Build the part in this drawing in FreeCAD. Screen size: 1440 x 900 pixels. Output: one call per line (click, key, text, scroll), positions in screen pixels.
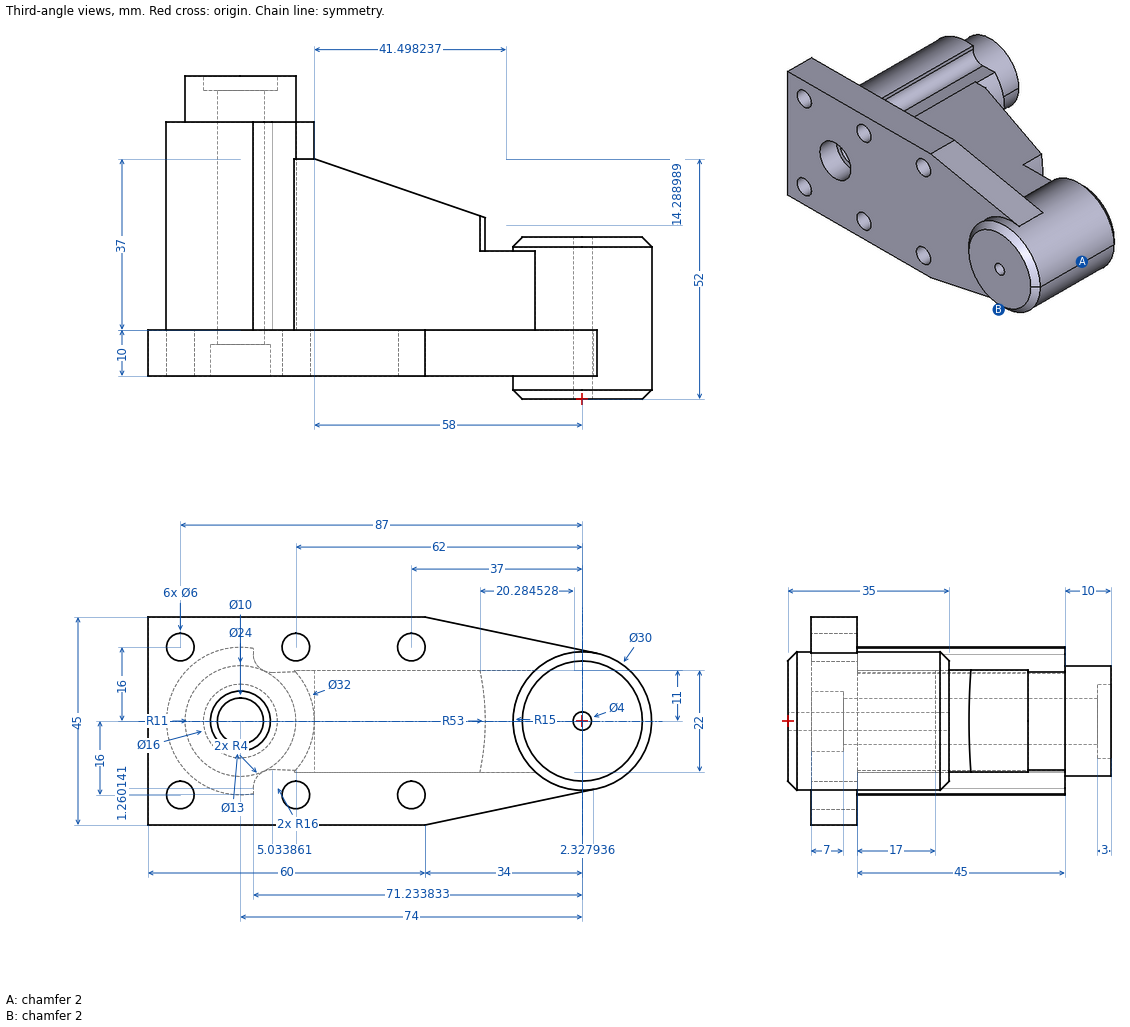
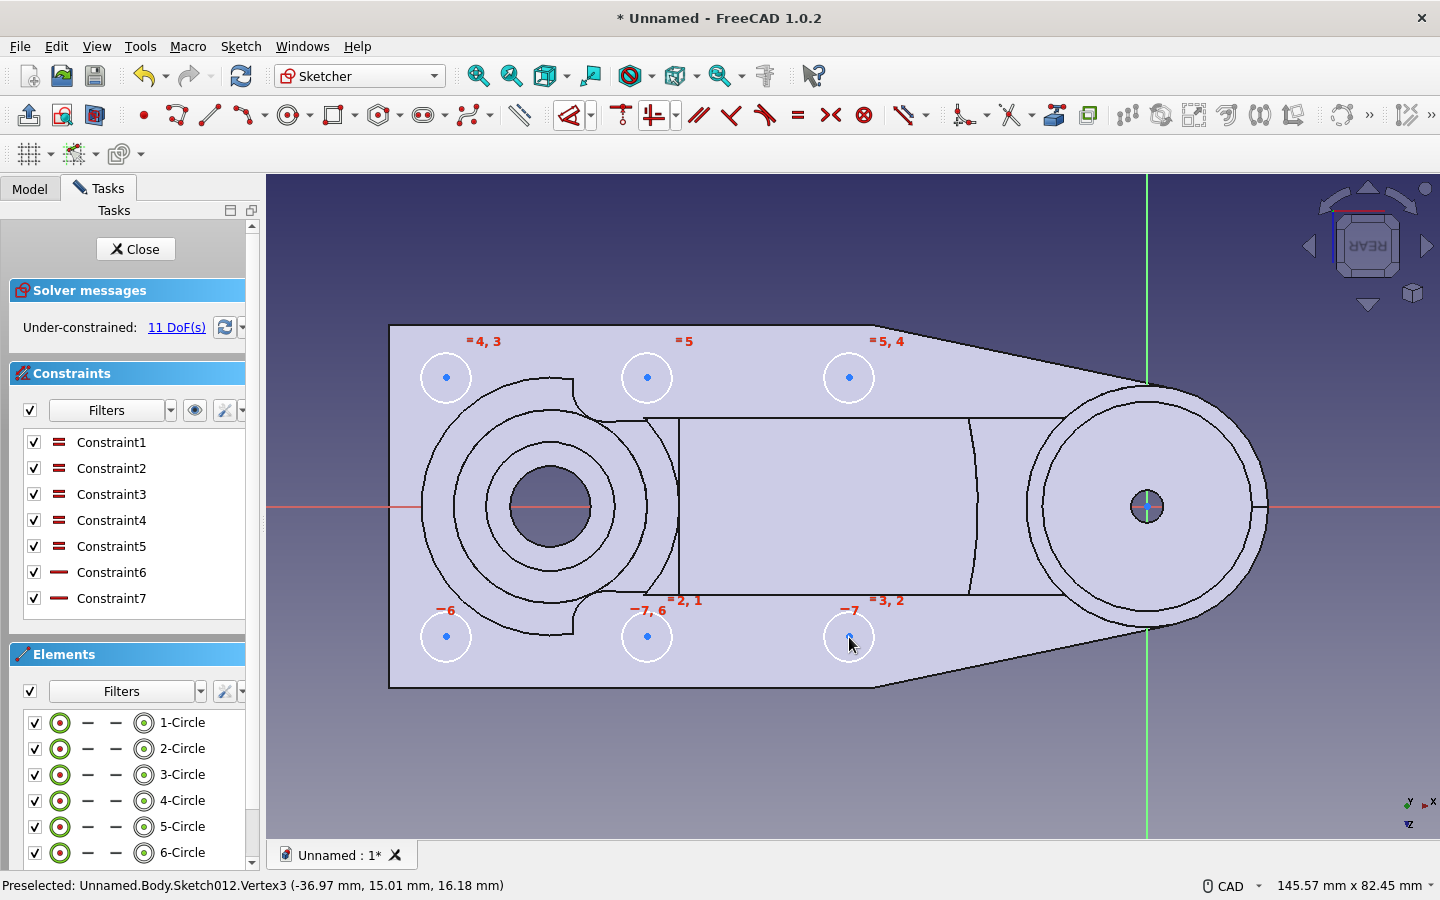
click(446, 637)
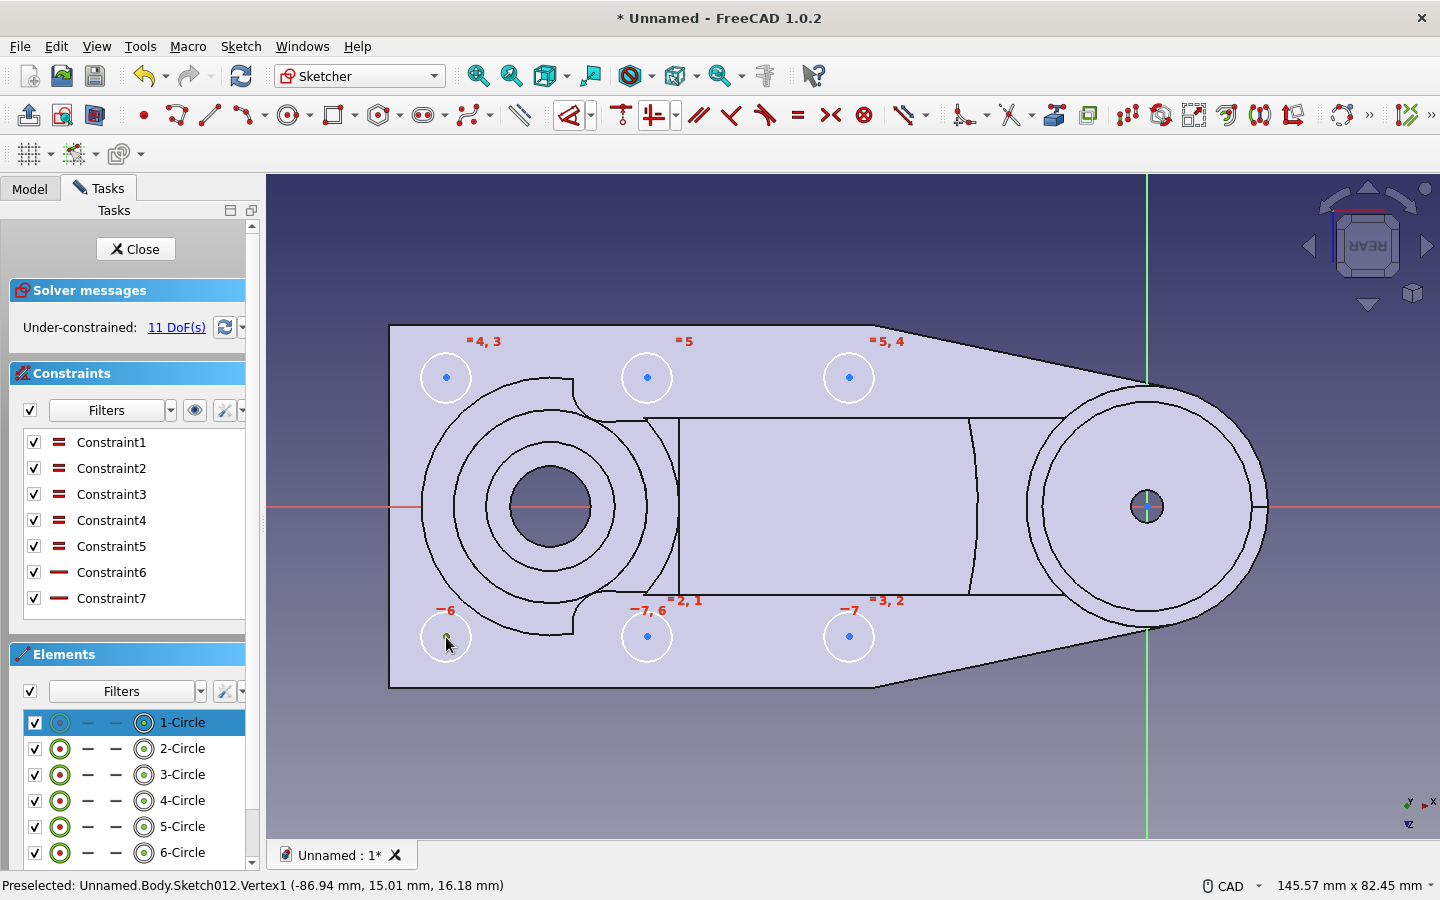
click(446, 378)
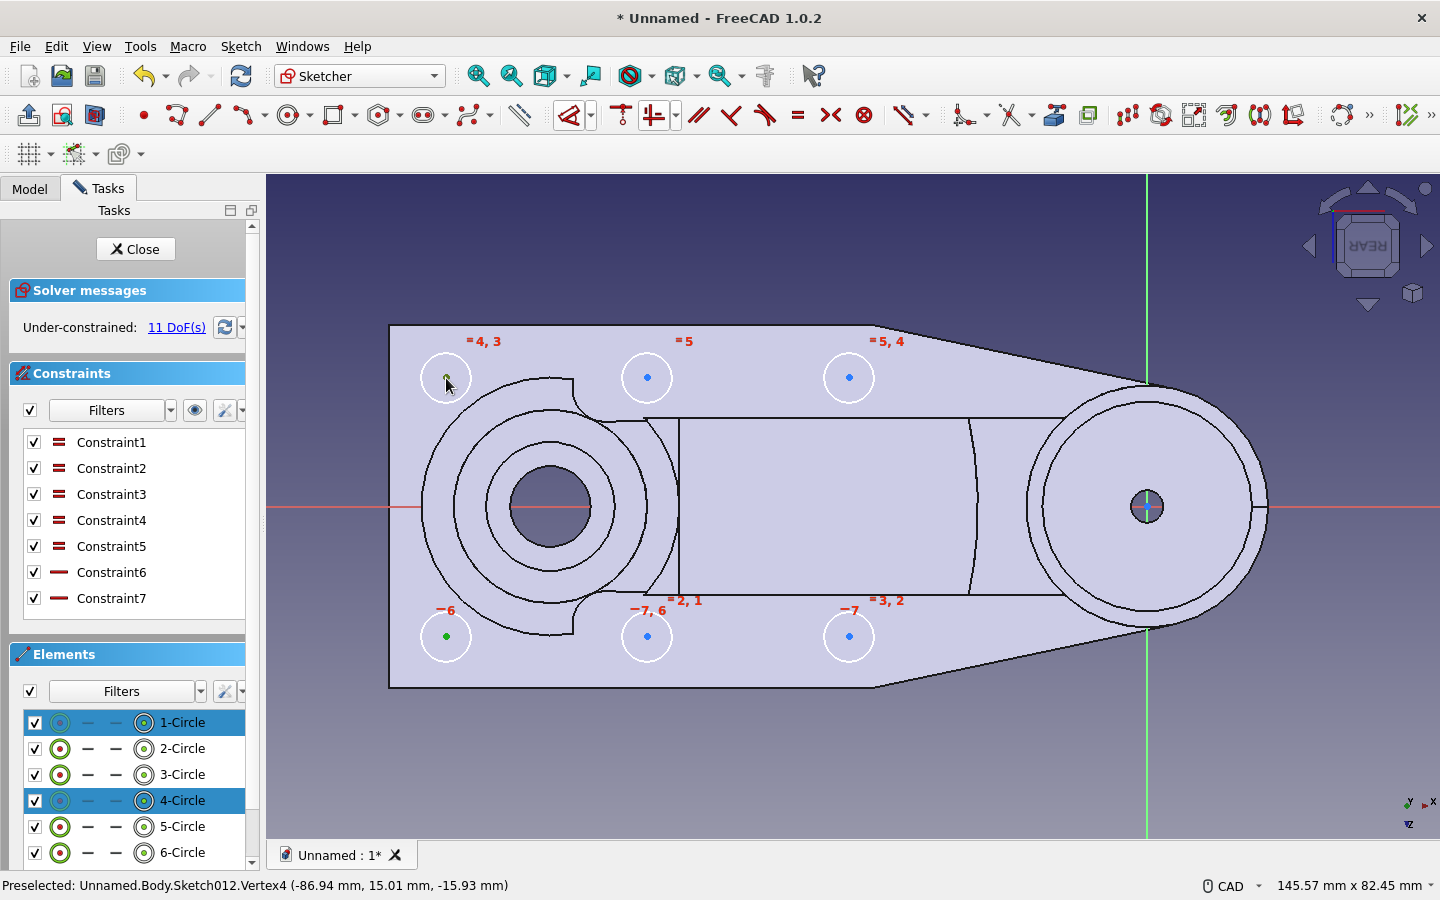
click(676, 116)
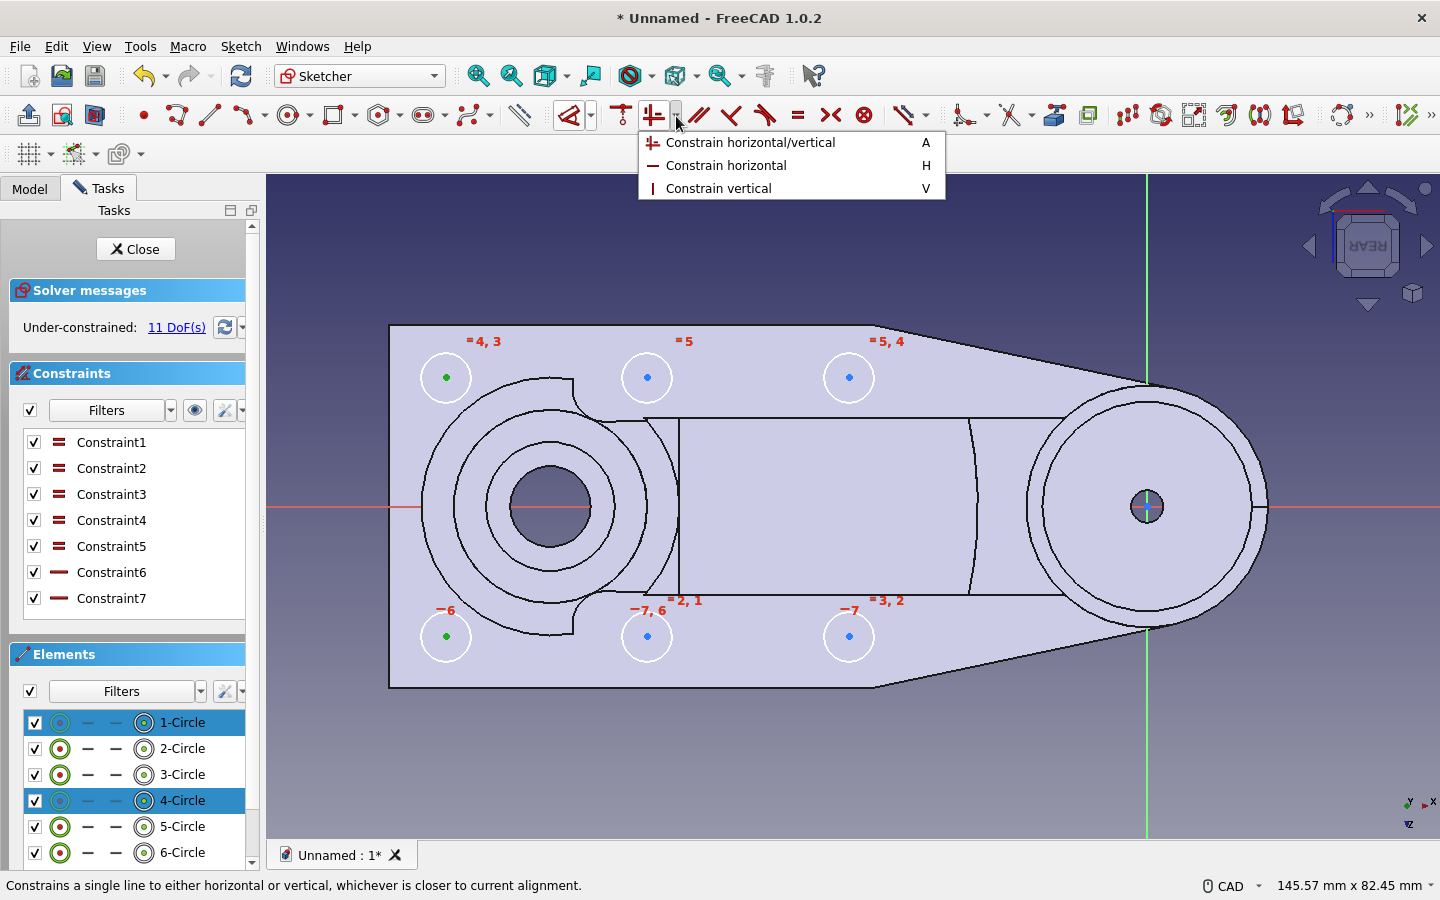
click(792, 188)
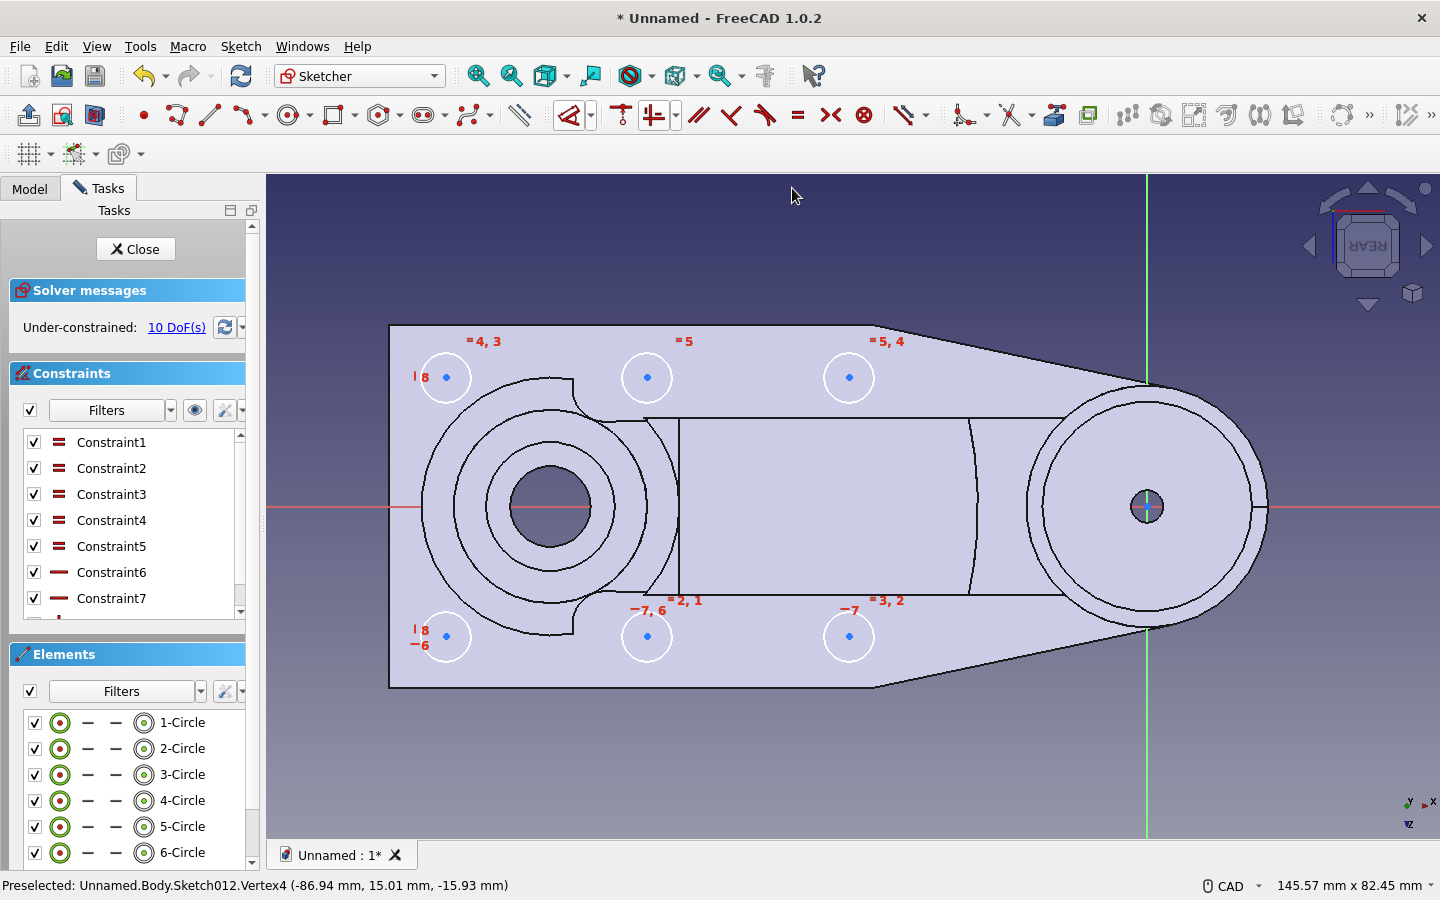
click(849, 637)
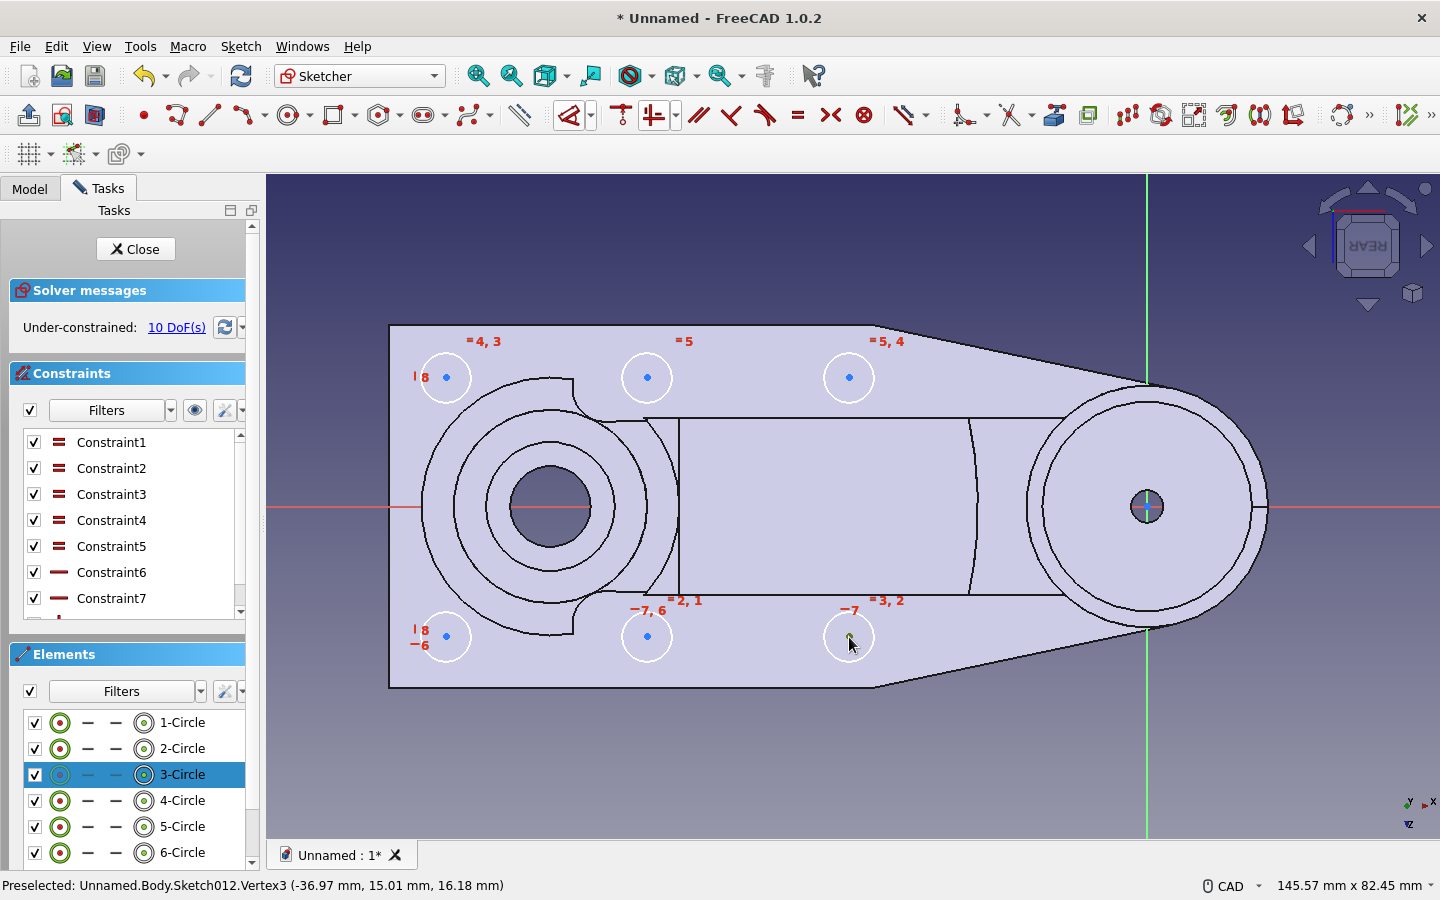
click(849, 378)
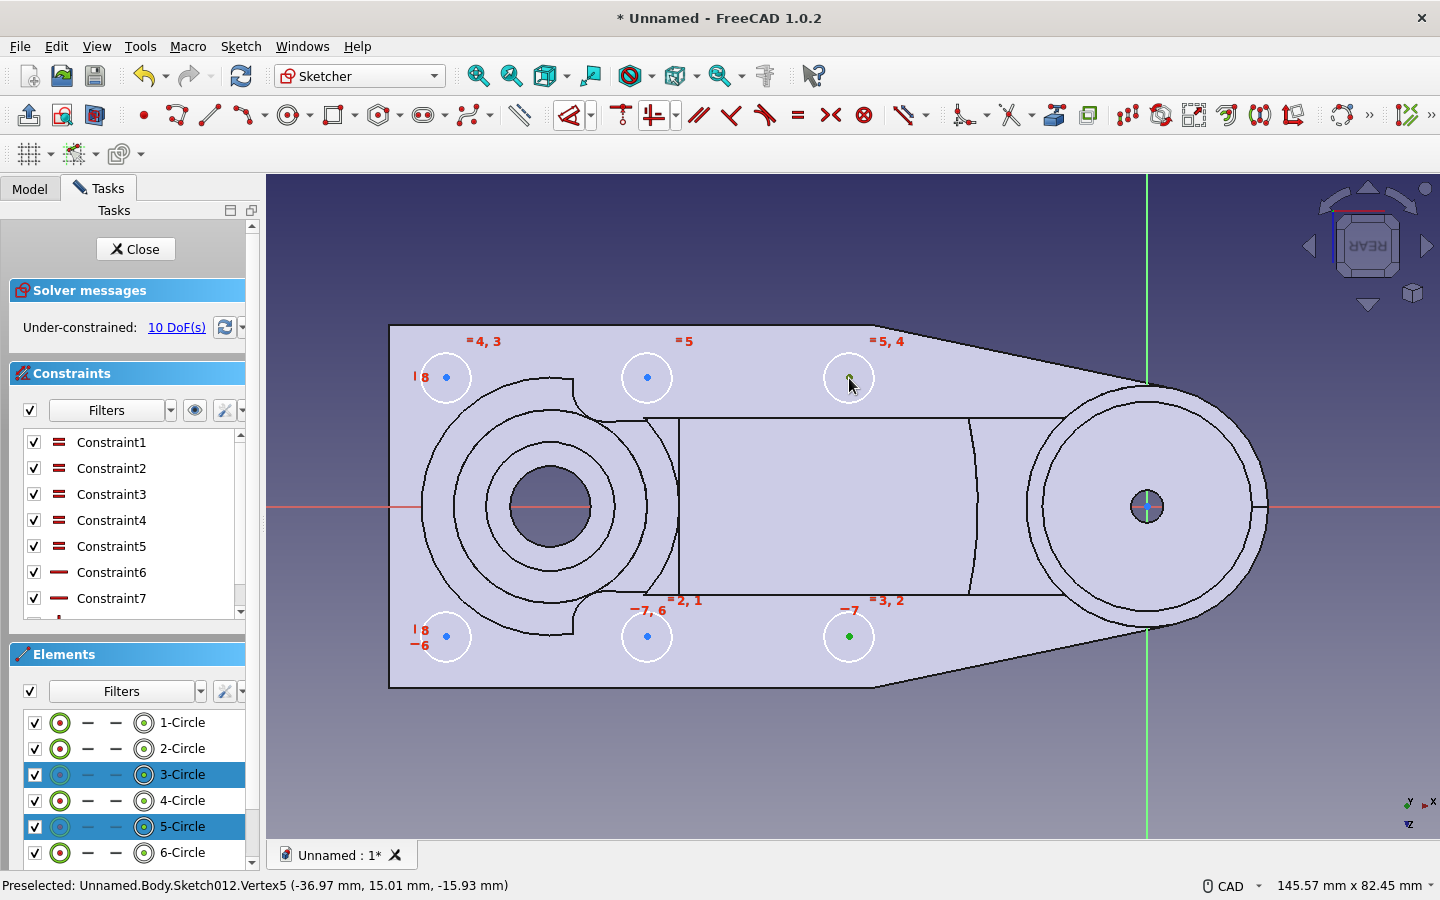
key(v)